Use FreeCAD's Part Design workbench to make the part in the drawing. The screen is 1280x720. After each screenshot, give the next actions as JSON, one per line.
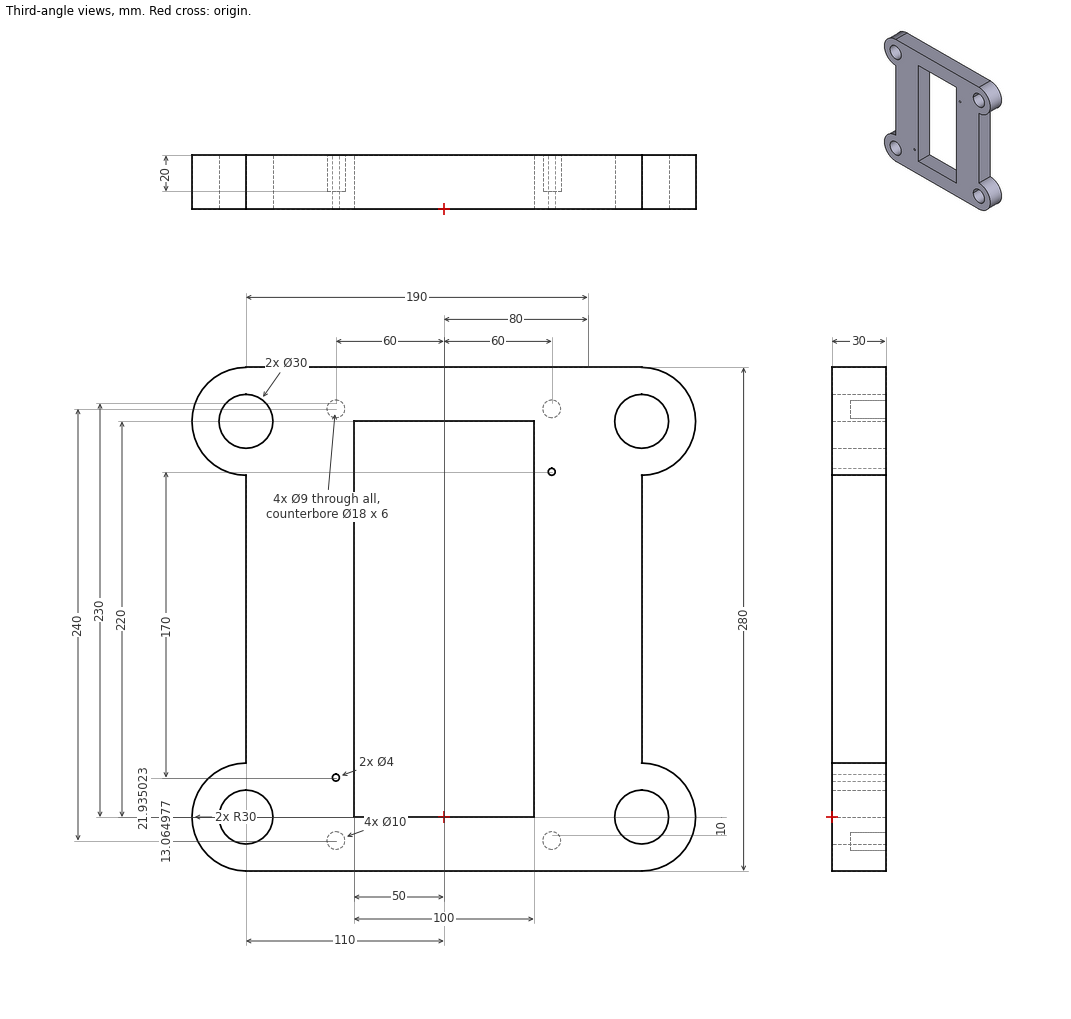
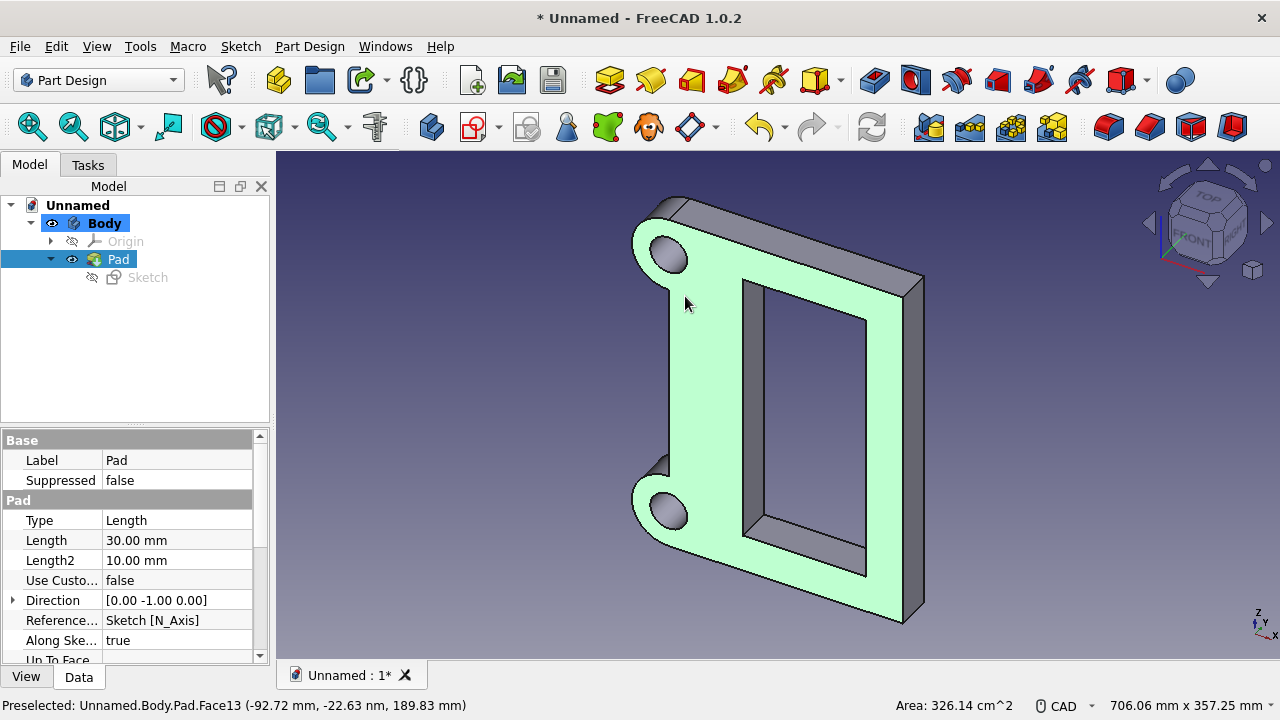
{"action": "left_click", "coordinate": [472, 128]}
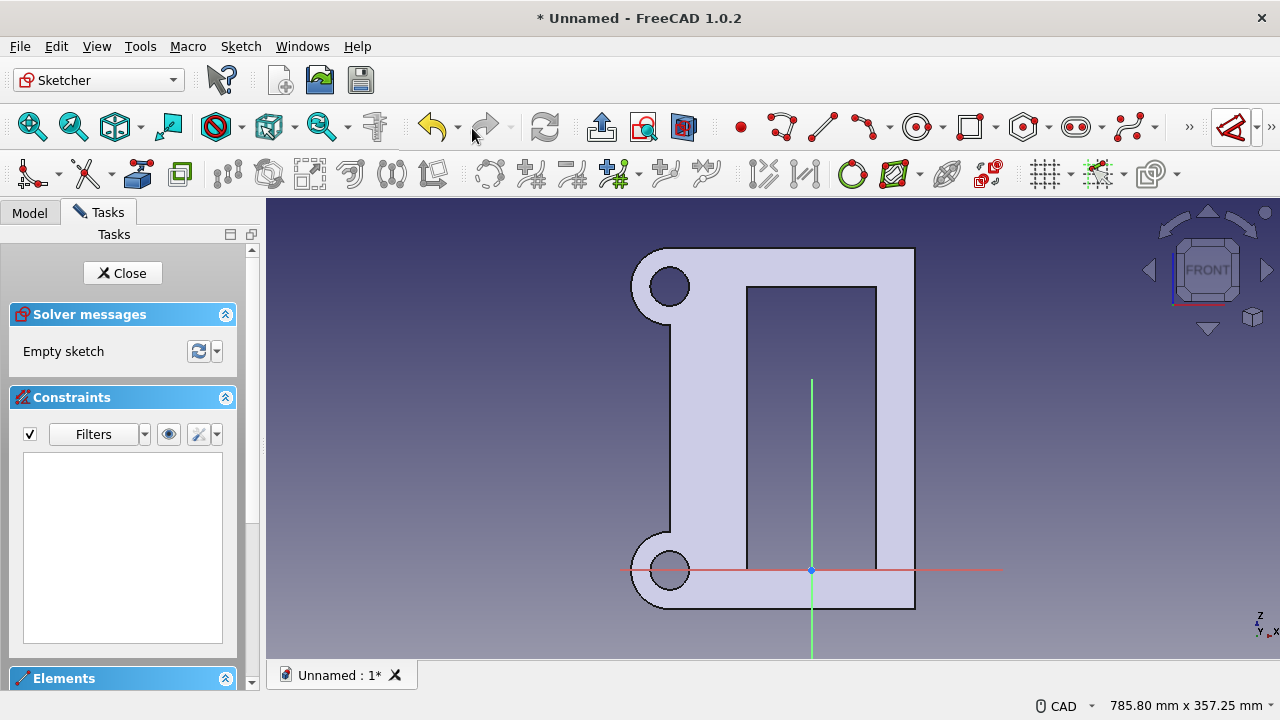
{"action": "key", "text": "g c"}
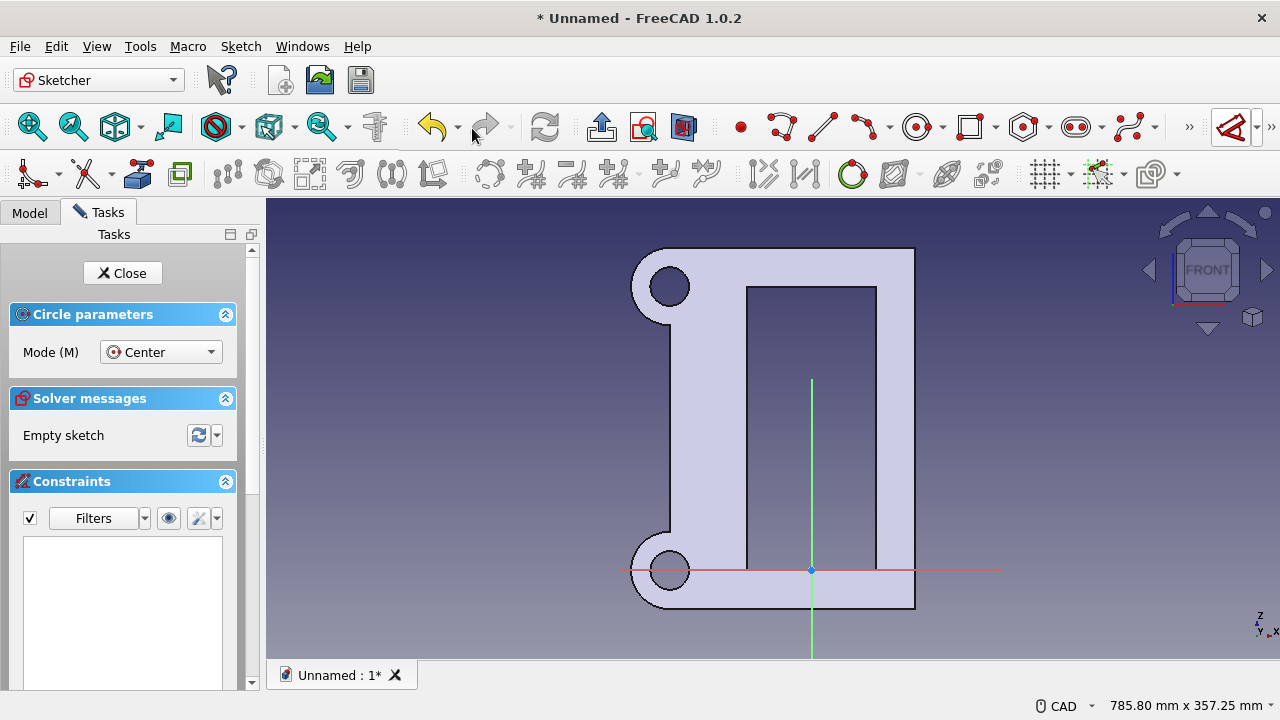
{"action": "scroll", "coordinate": [734, 274], "scroll_direction": "up", "scroll_amount": 7}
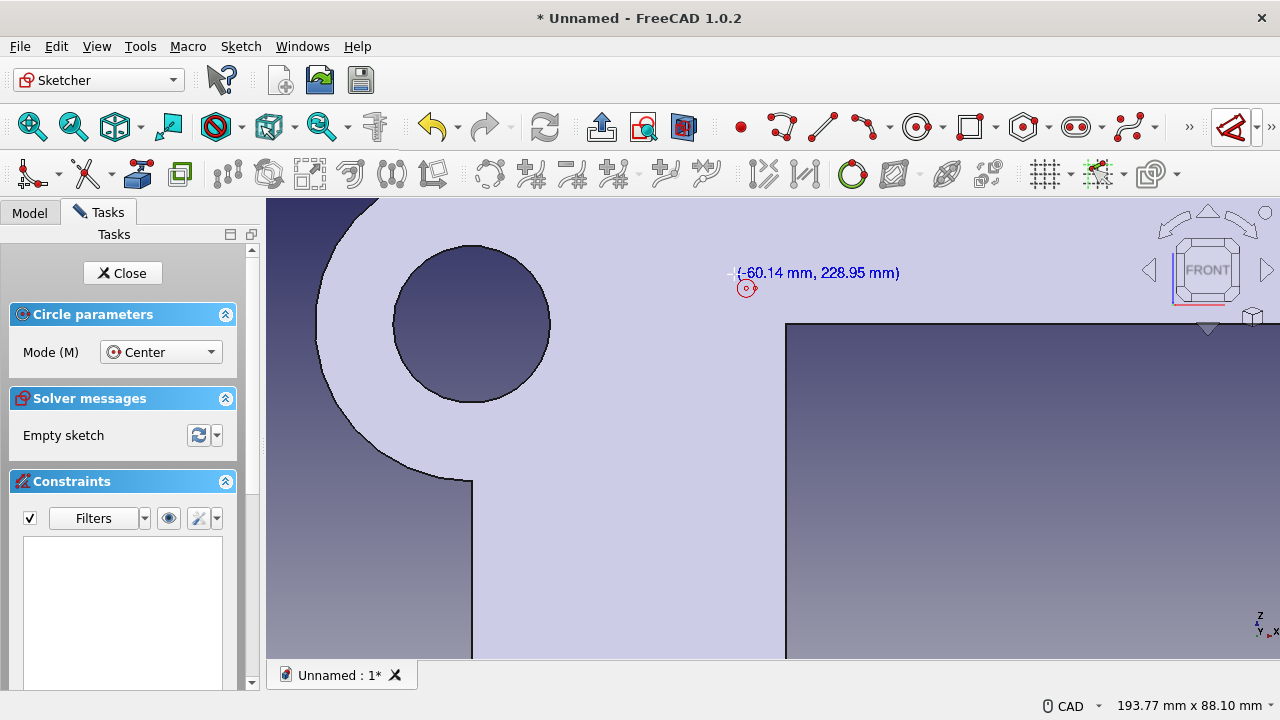
{"action": "scroll", "coordinate": [618, 309], "scroll_direction": "down", "scroll_amount": 8}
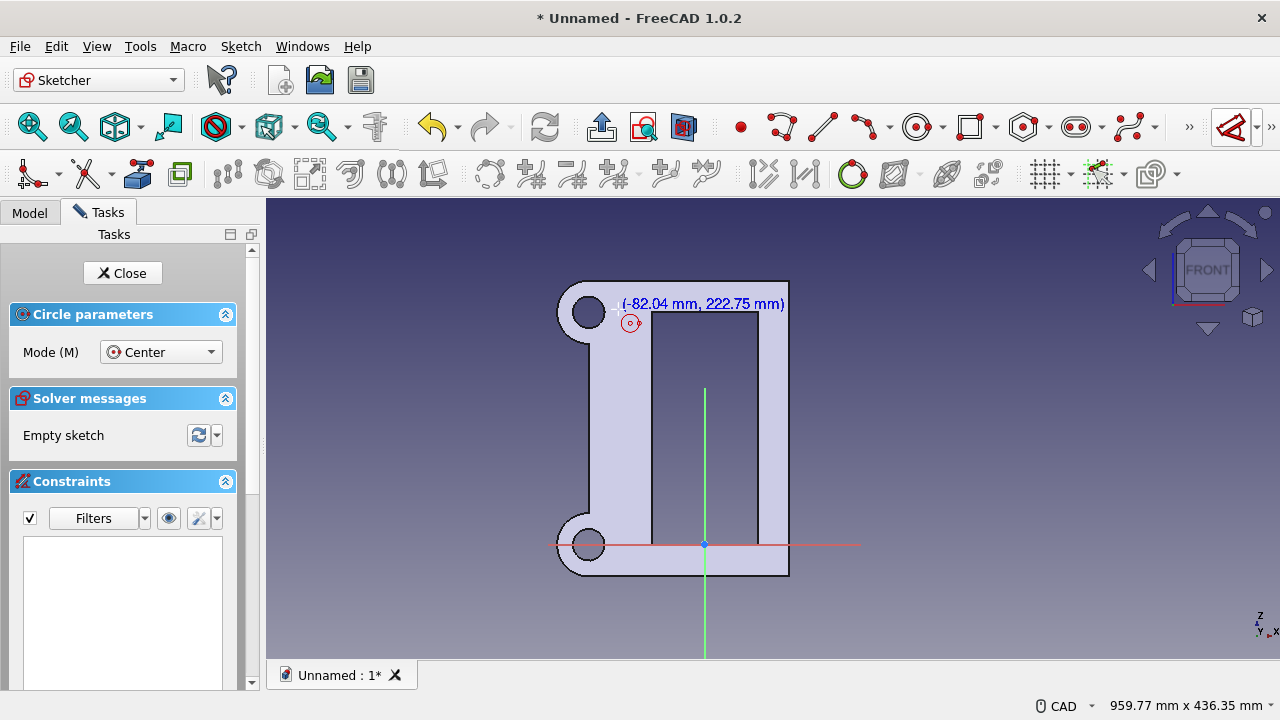
{"action": "left_click", "coordinate": [642, 302]}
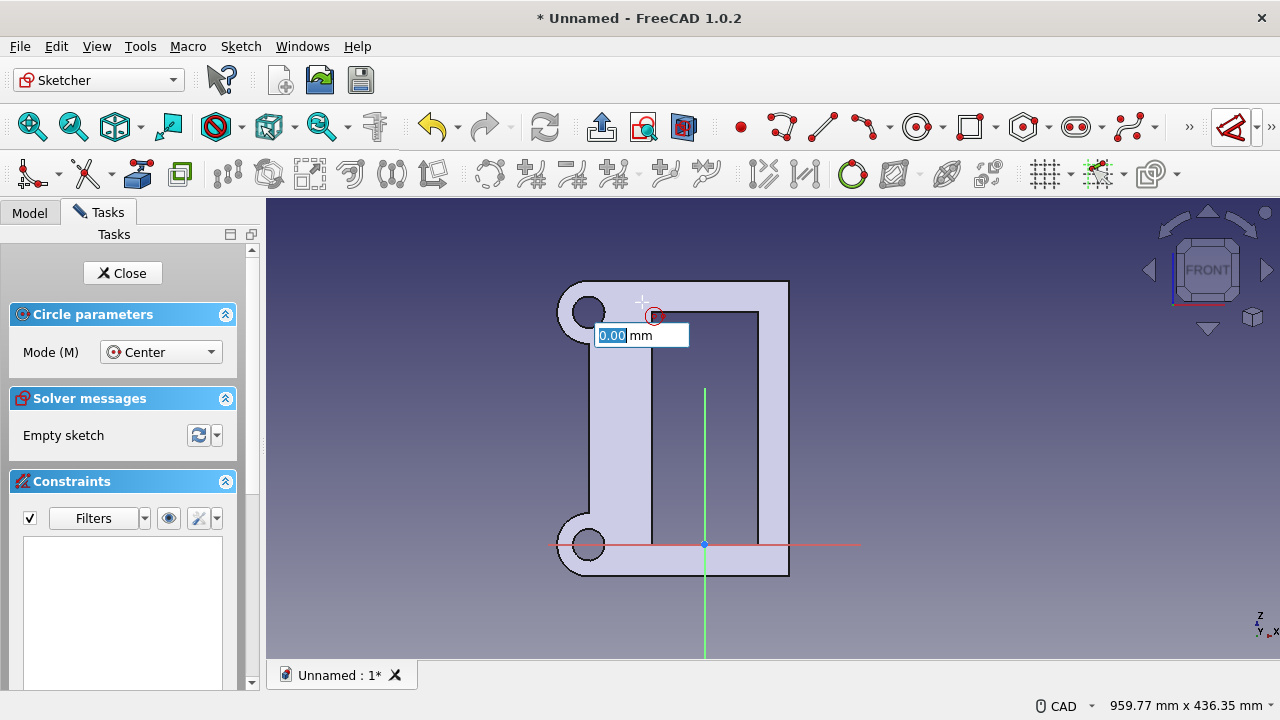
{"action": "scroll", "coordinate": [645, 298], "scroll_direction": "up", "scroll_amount": 7}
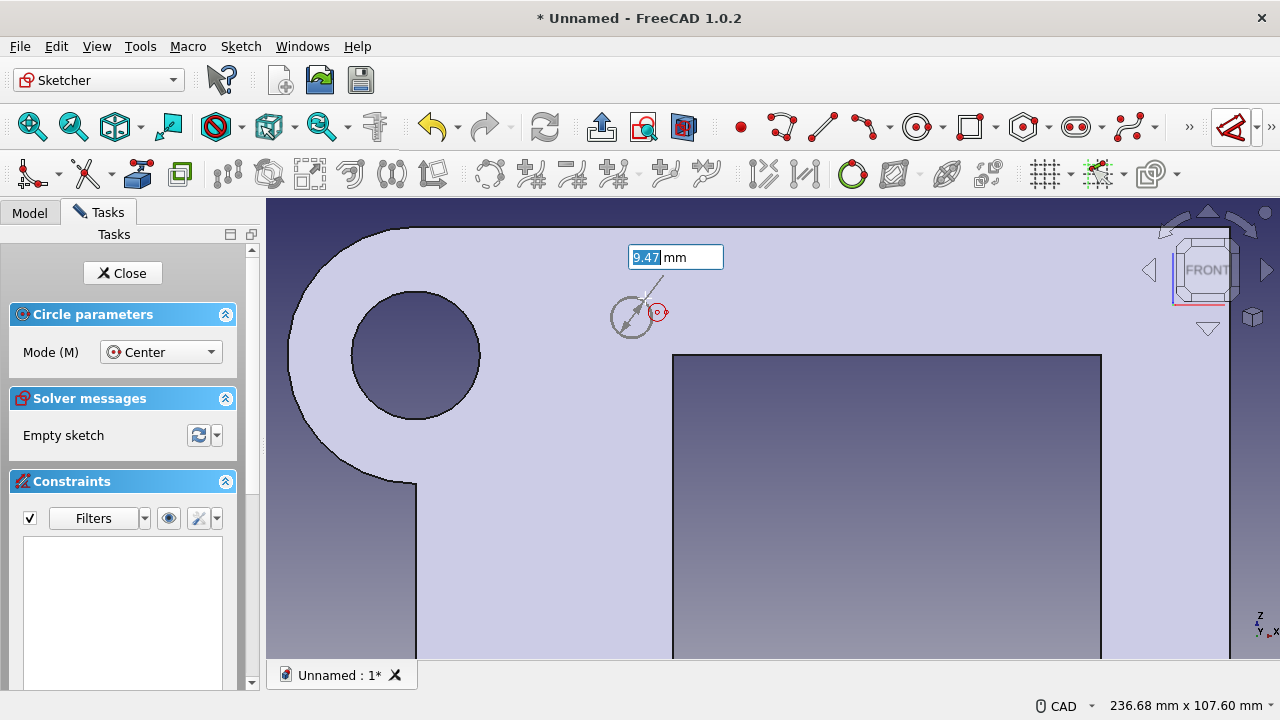
{"action": "left_click", "coordinate": [644, 299]}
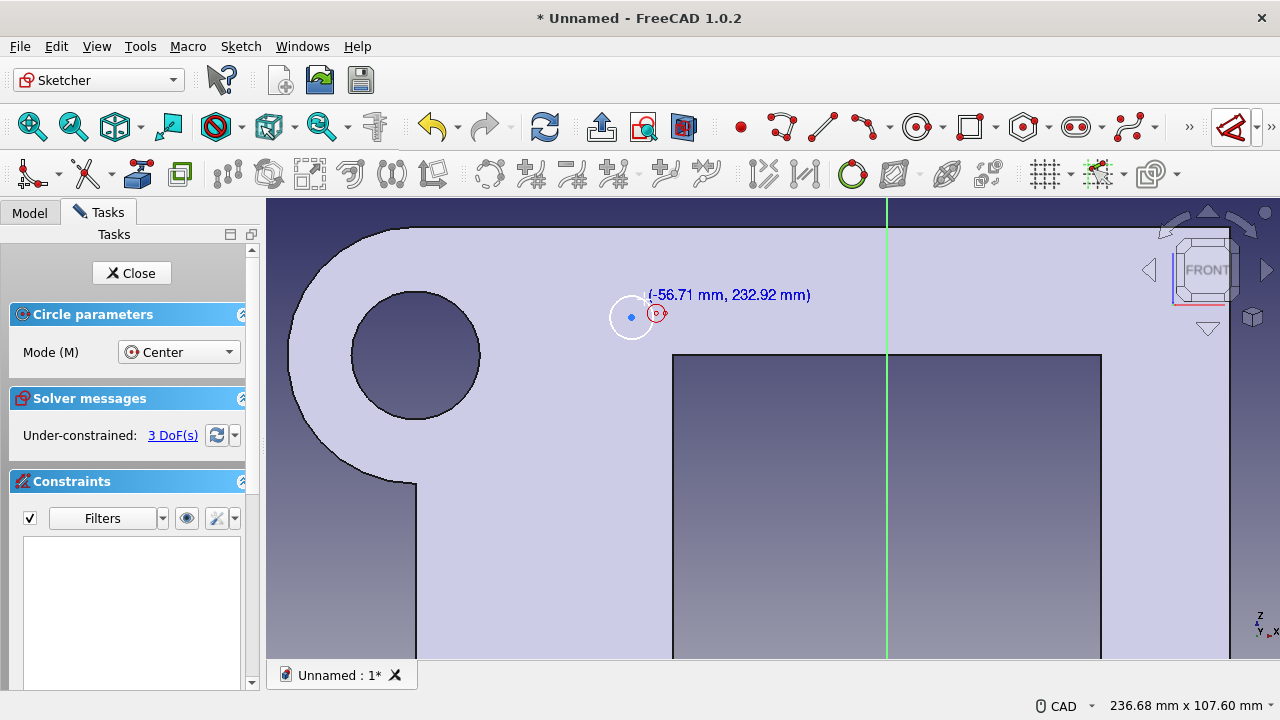
{"action": "scroll", "coordinate": [645, 298], "scroll_direction": "down", "scroll_amount": 7}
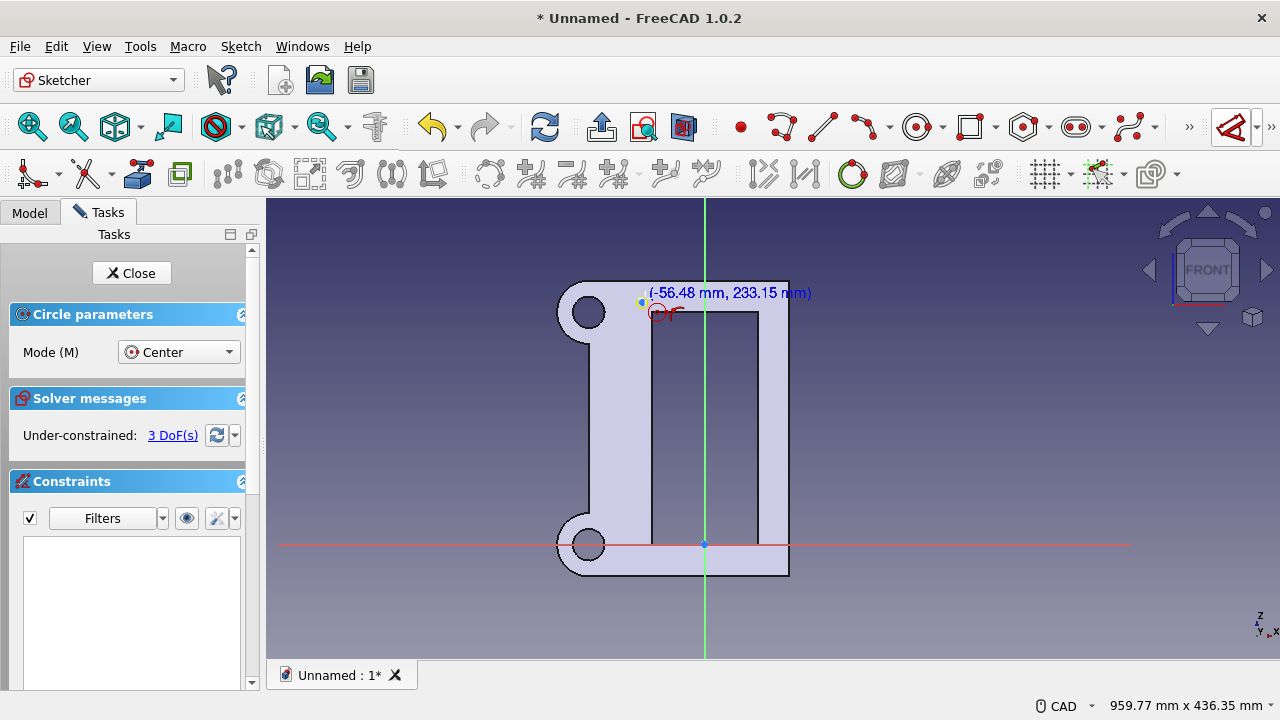
{"action": "scroll", "coordinate": [768, 302], "scroll_direction": "up", "scroll_amount": 8}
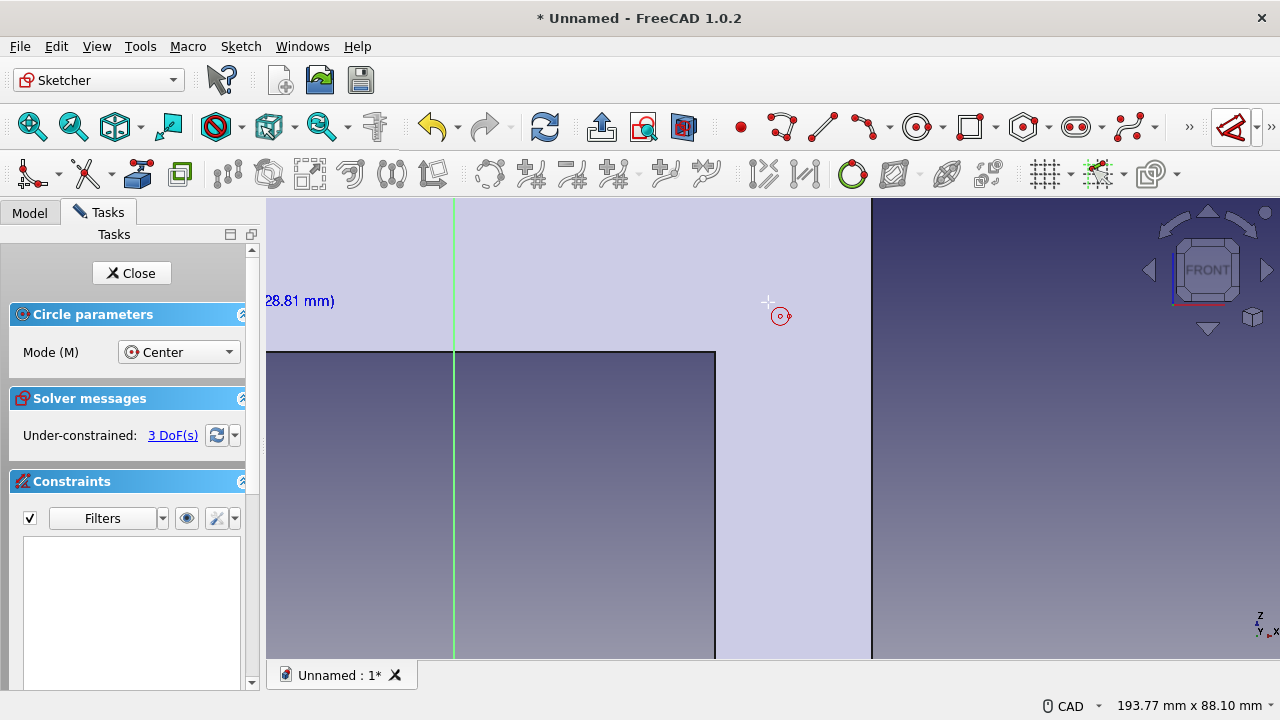
{"action": "scroll", "coordinate": [768, 302], "scroll_direction": "down", "scroll_amount": 8}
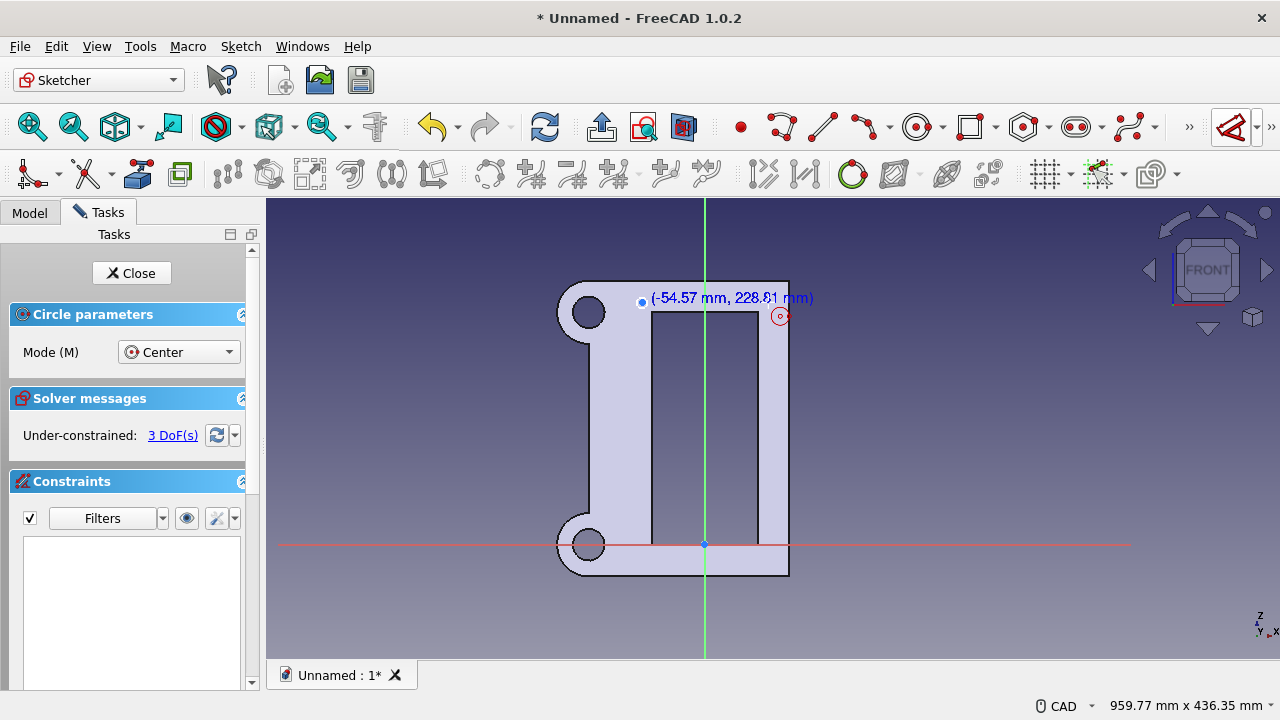
{"action": "left_click", "coordinate": [768, 302]}